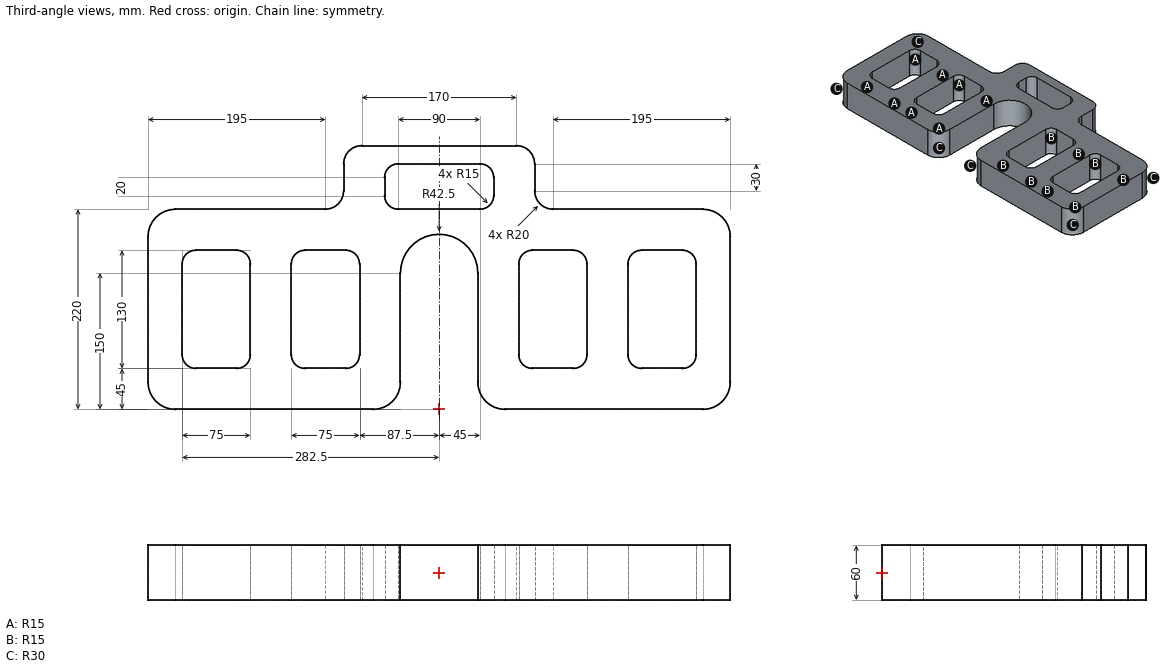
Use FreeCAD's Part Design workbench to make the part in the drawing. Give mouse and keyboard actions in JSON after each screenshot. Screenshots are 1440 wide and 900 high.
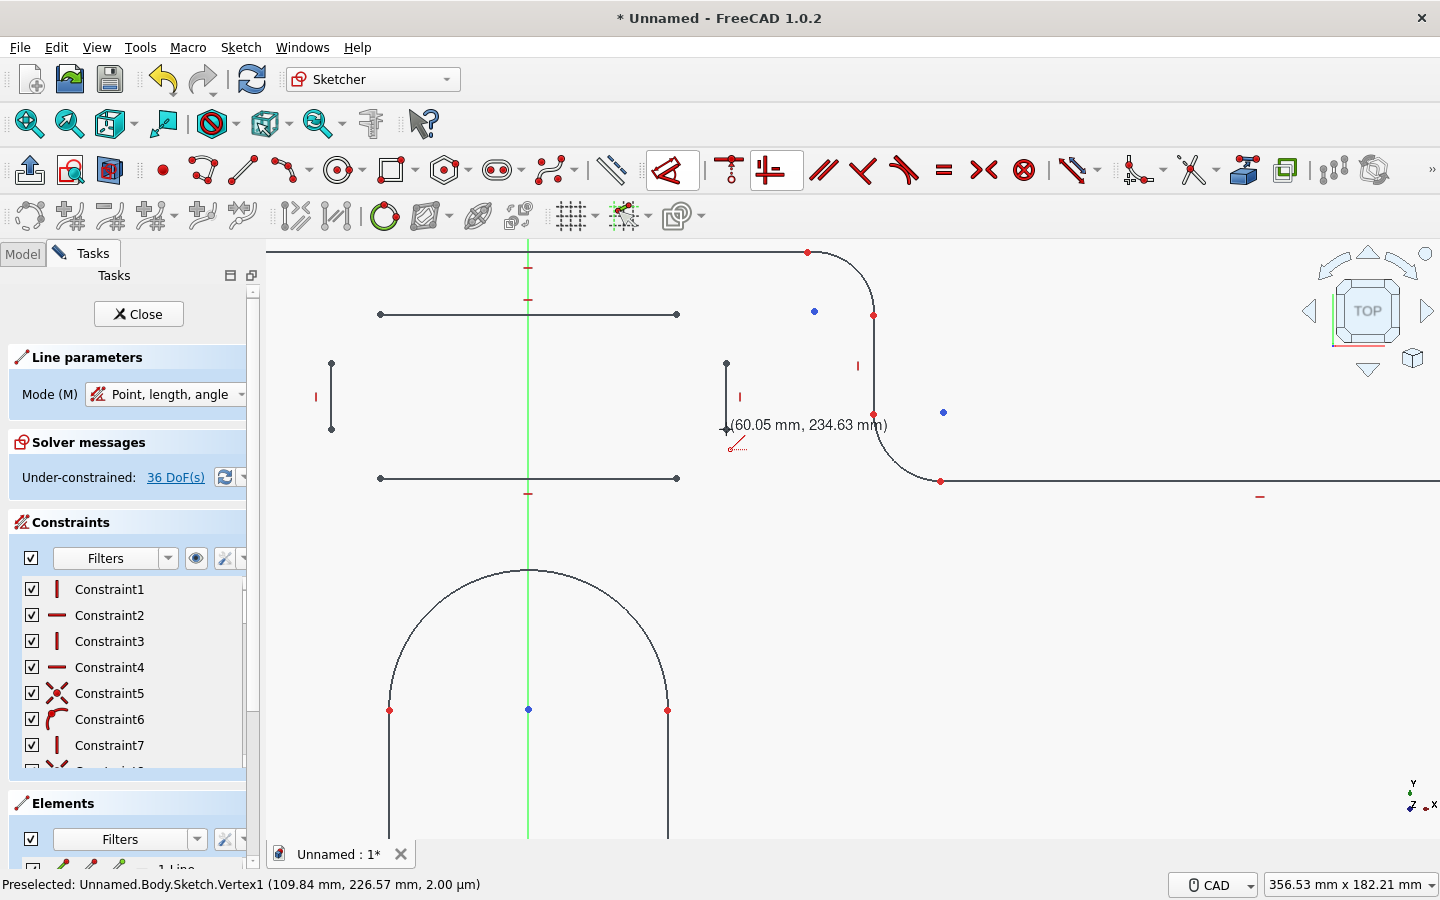
{"action": "left_click", "coordinate": [284, 170]}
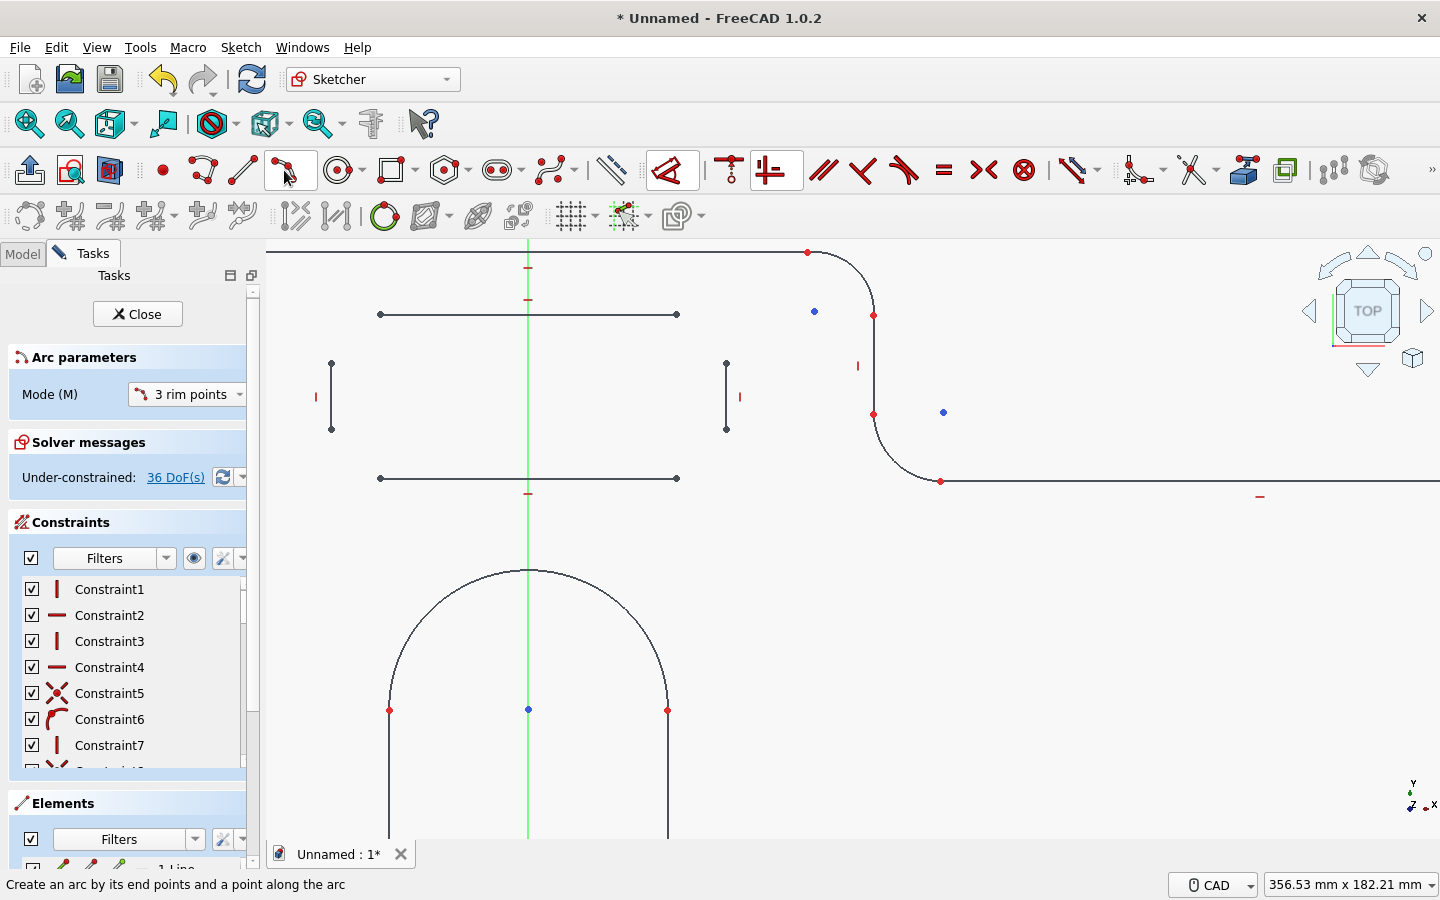
{"action": "left_click", "coordinate": [380, 479]}
{"action": "left_click", "coordinate": [331, 430]}
{"action": "left_click", "coordinate": [345, 464]}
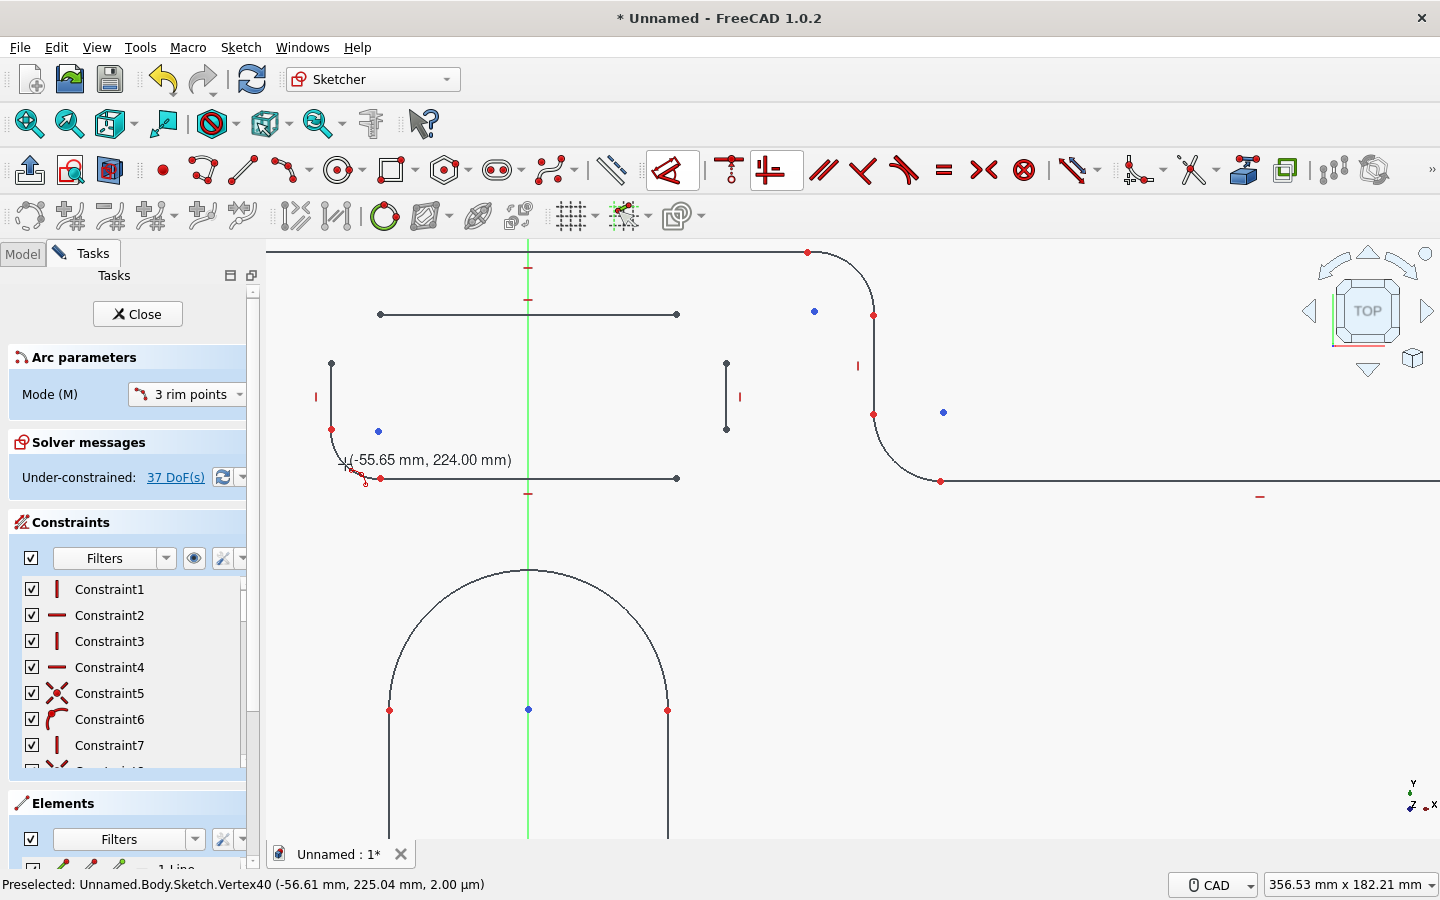
{"action": "left_click", "coordinate": [331, 364]}
{"action": "left_click", "coordinate": [380, 315]}
{"action": "left_click", "coordinate": [345, 328]}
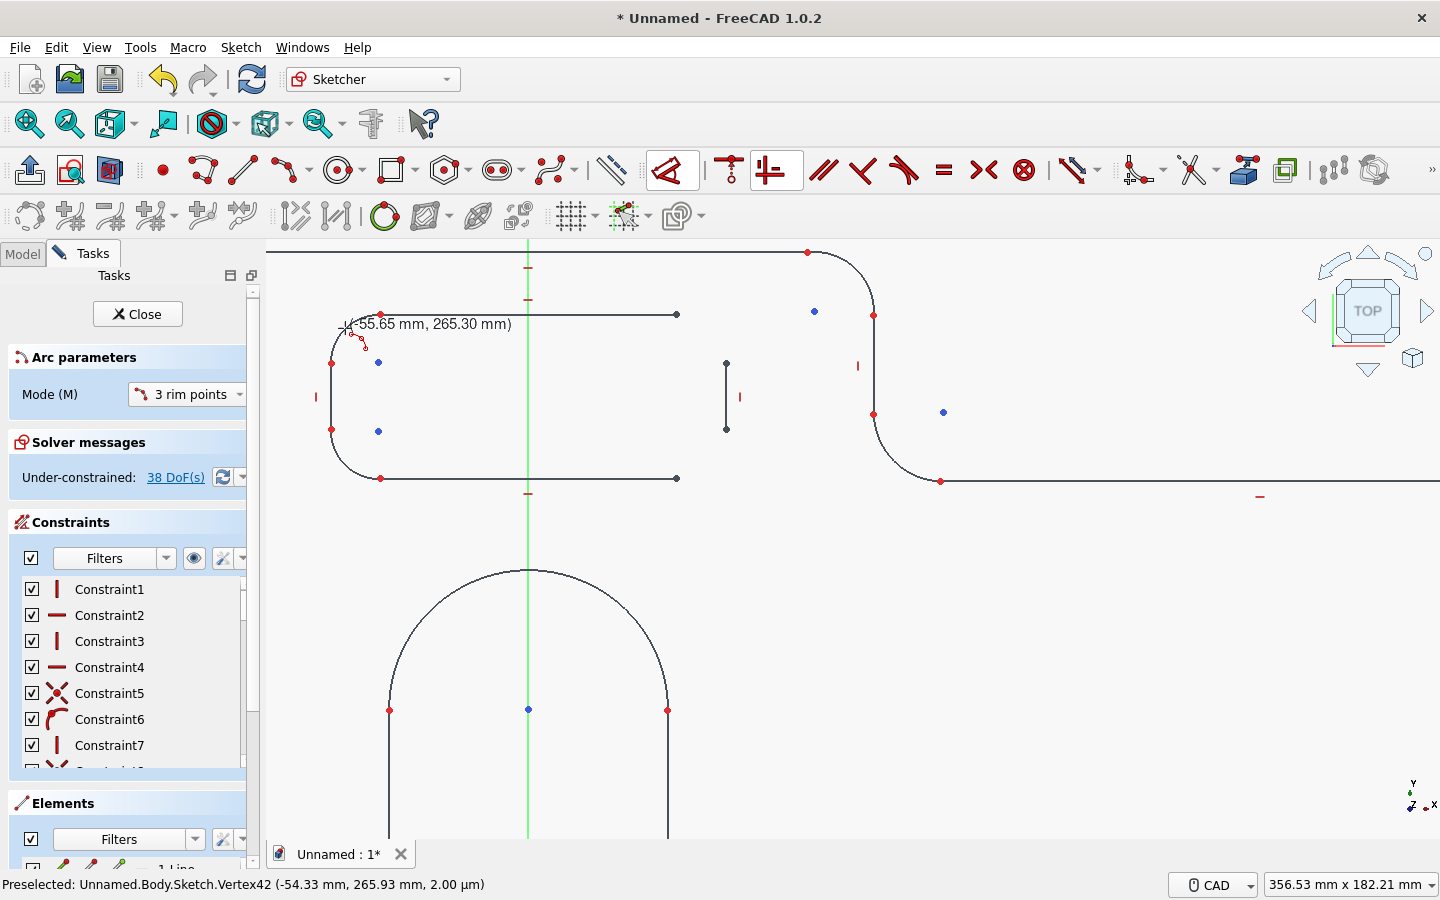
{"action": "left_click", "coordinate": [676, 315]}
{"action": "left_click", "coordinate": [726, 364]}
{"action": "left_click", "coordinate": [711, 328]}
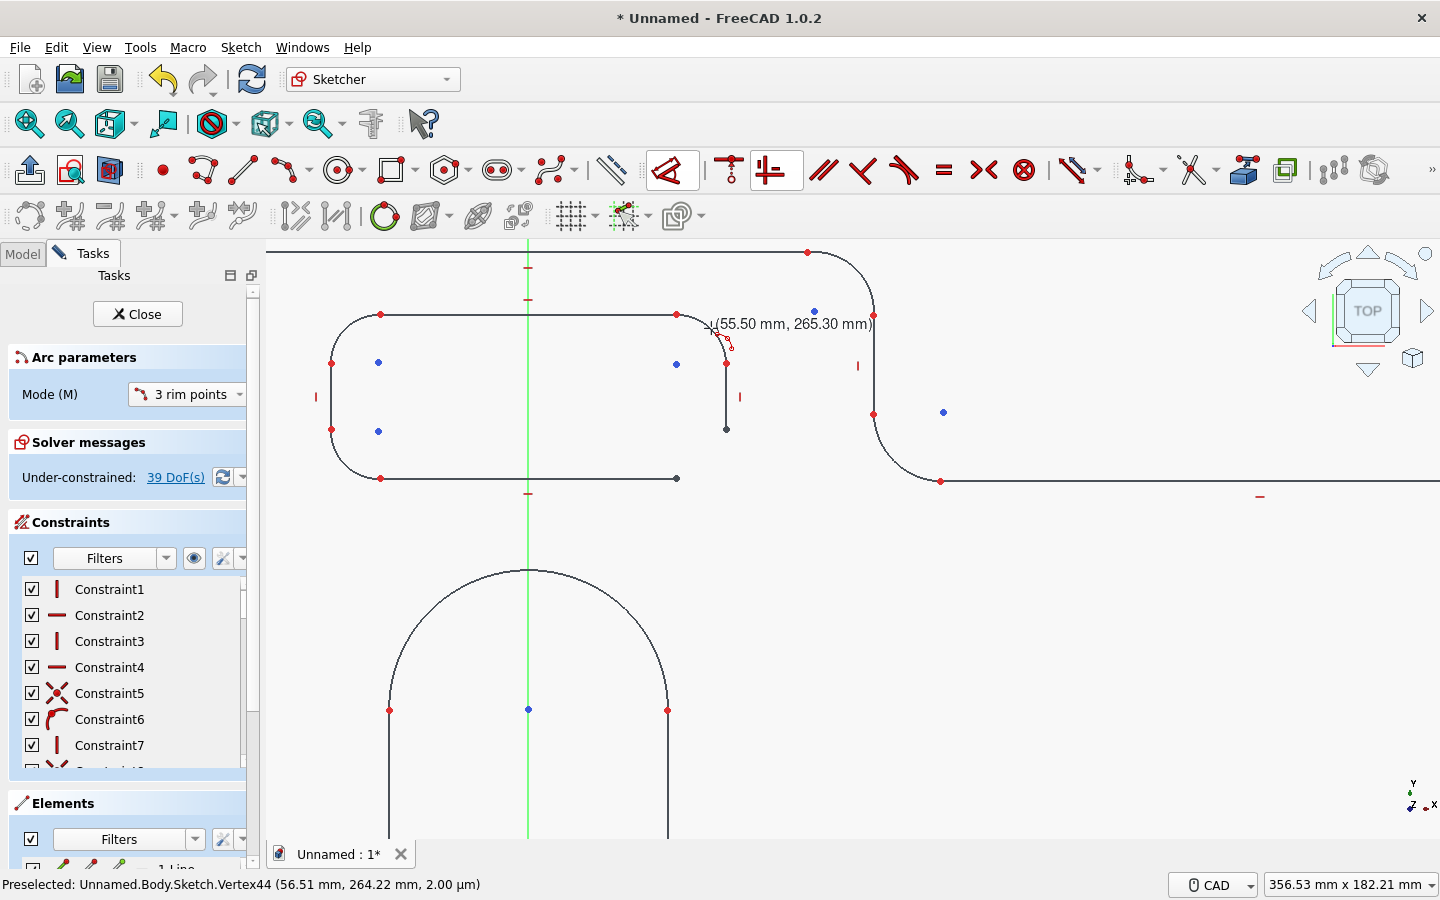
{"action": "left_click", "coordinate": [726, 430]}
{"action": "left_click", "coordinate": [676, 479]}
{"action": "left_click", "coordinate": [711, 464]}
{"action": "key", "text": "Escape"}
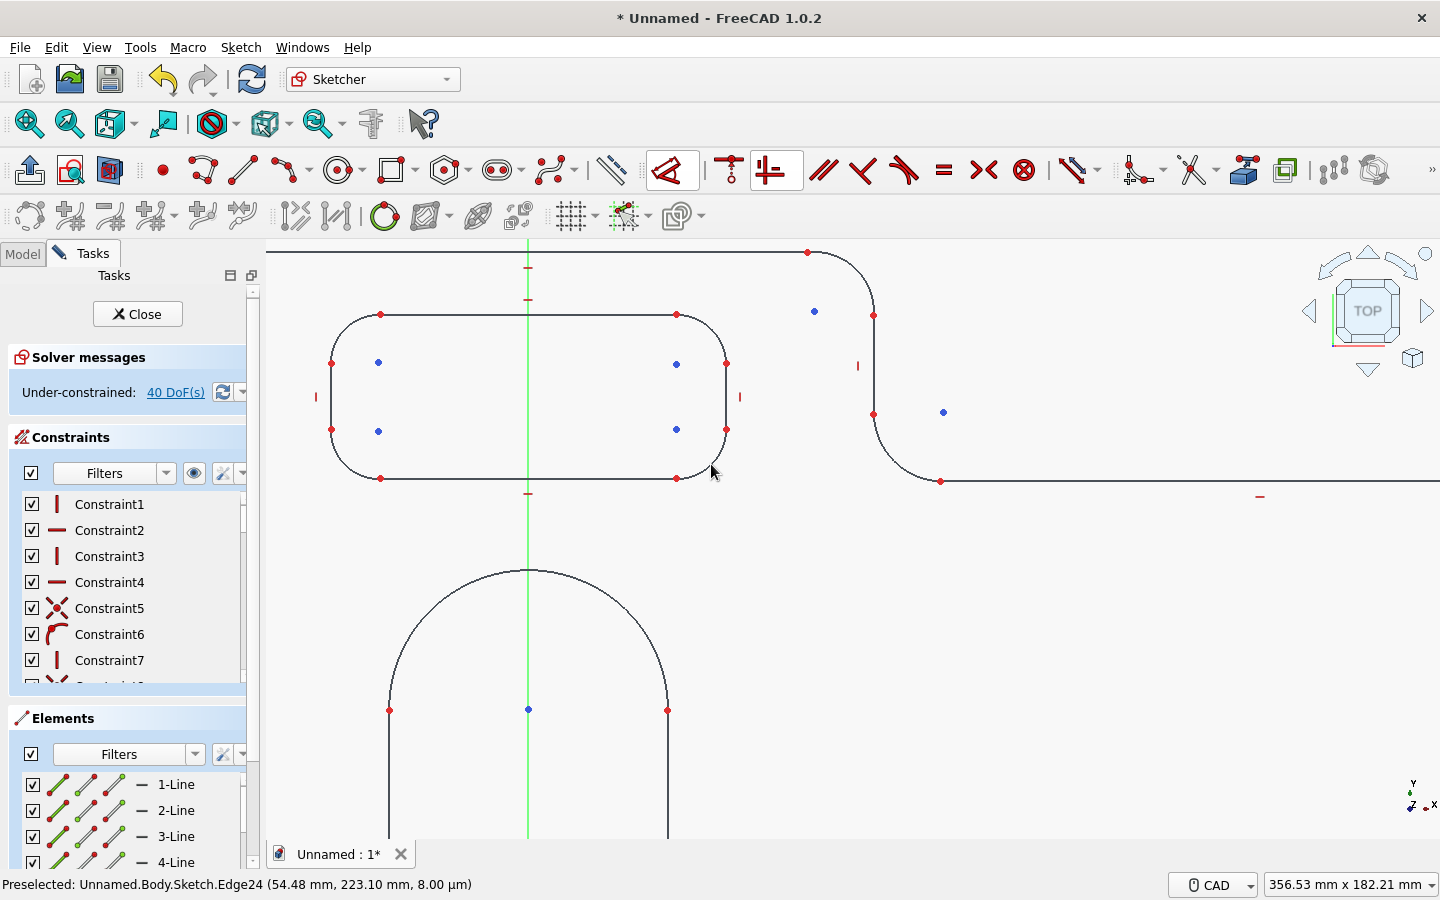
{"action": "left_click", "coordinate": [874, 385]}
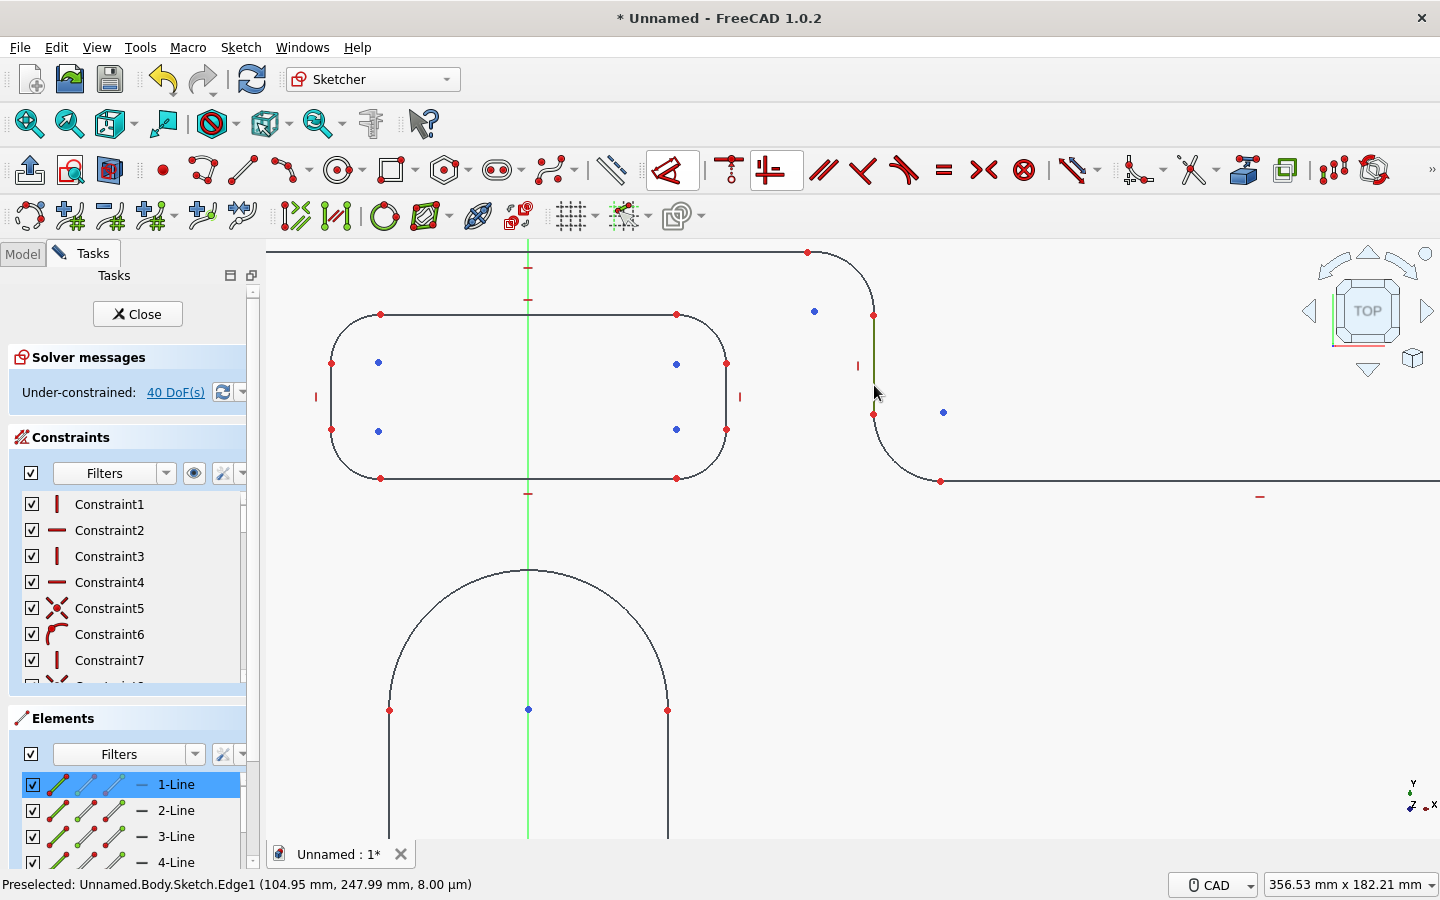
{"action": "left_click", "coordinate": [868, 285]}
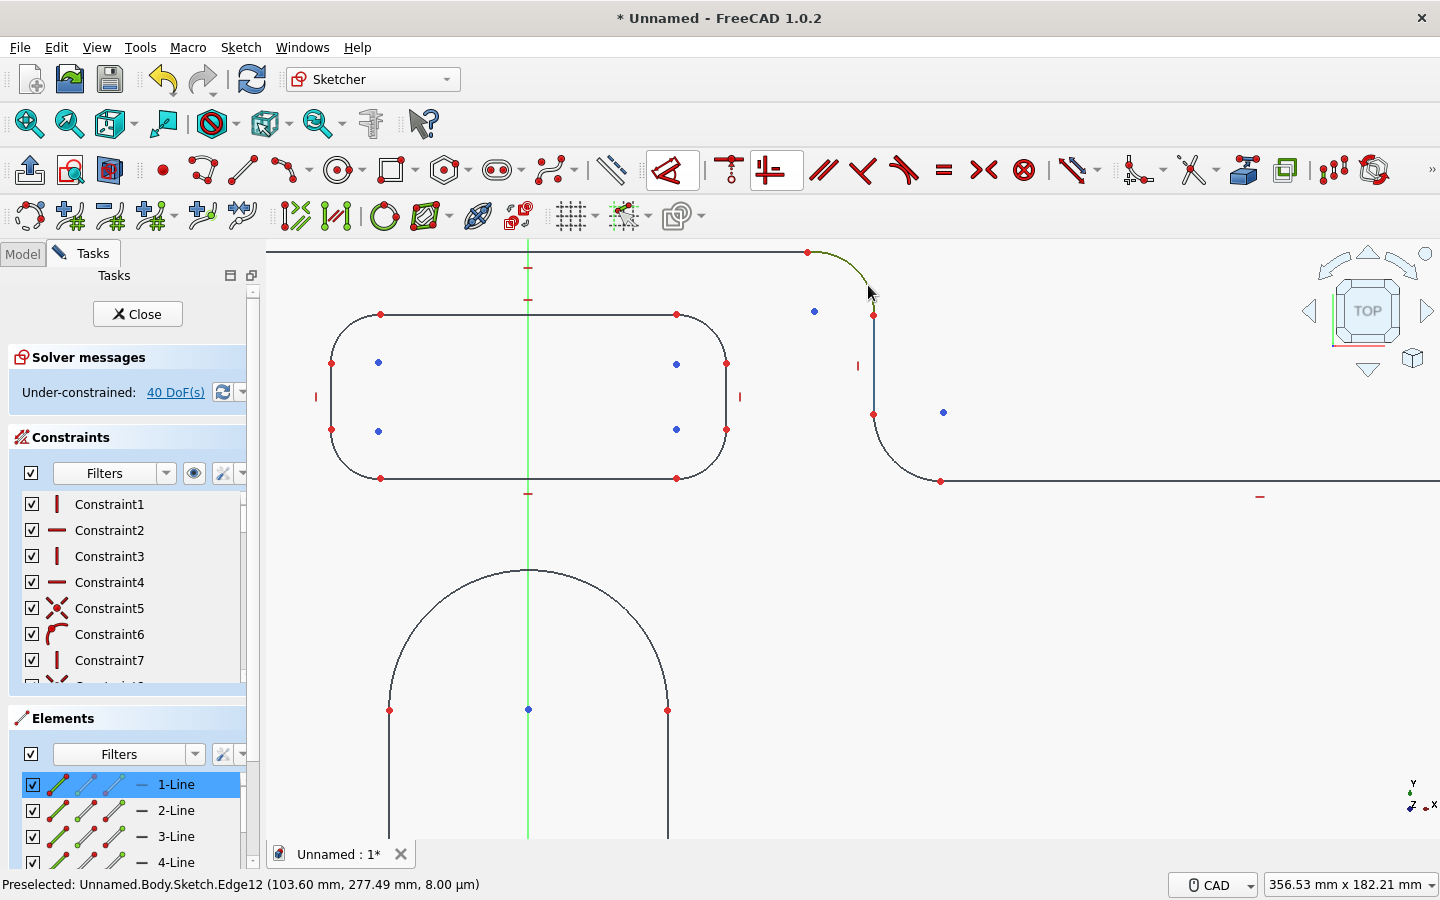
{"action": "key", "text": "t"}